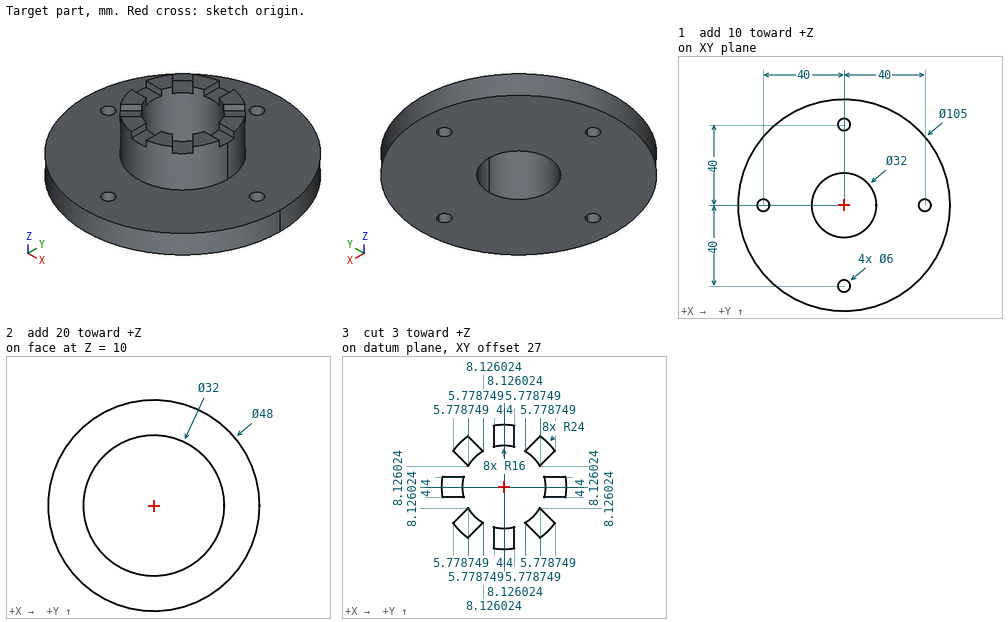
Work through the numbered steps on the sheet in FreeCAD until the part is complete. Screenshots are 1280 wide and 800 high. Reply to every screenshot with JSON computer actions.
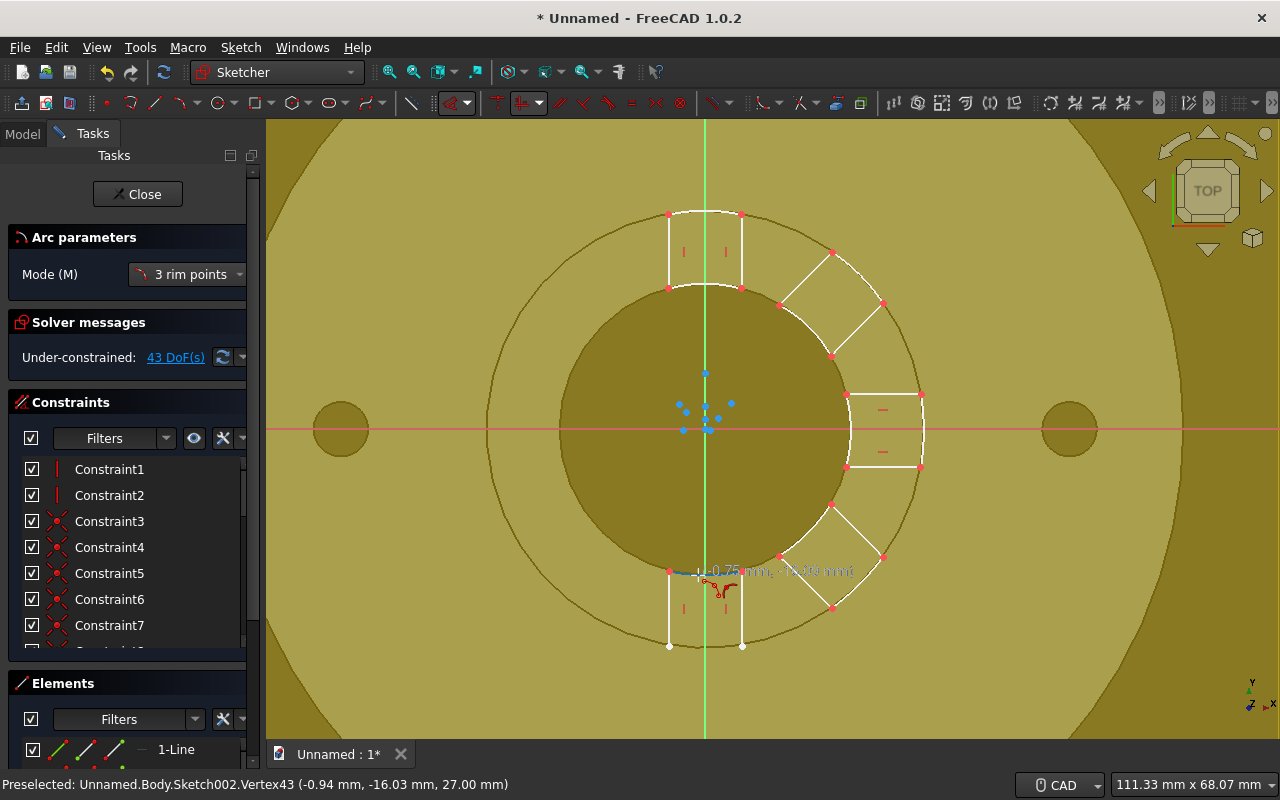
{"action": "left_click", "coordinate": [669, 646]}
{"action": "left_click", "coordinate": [742, 646]}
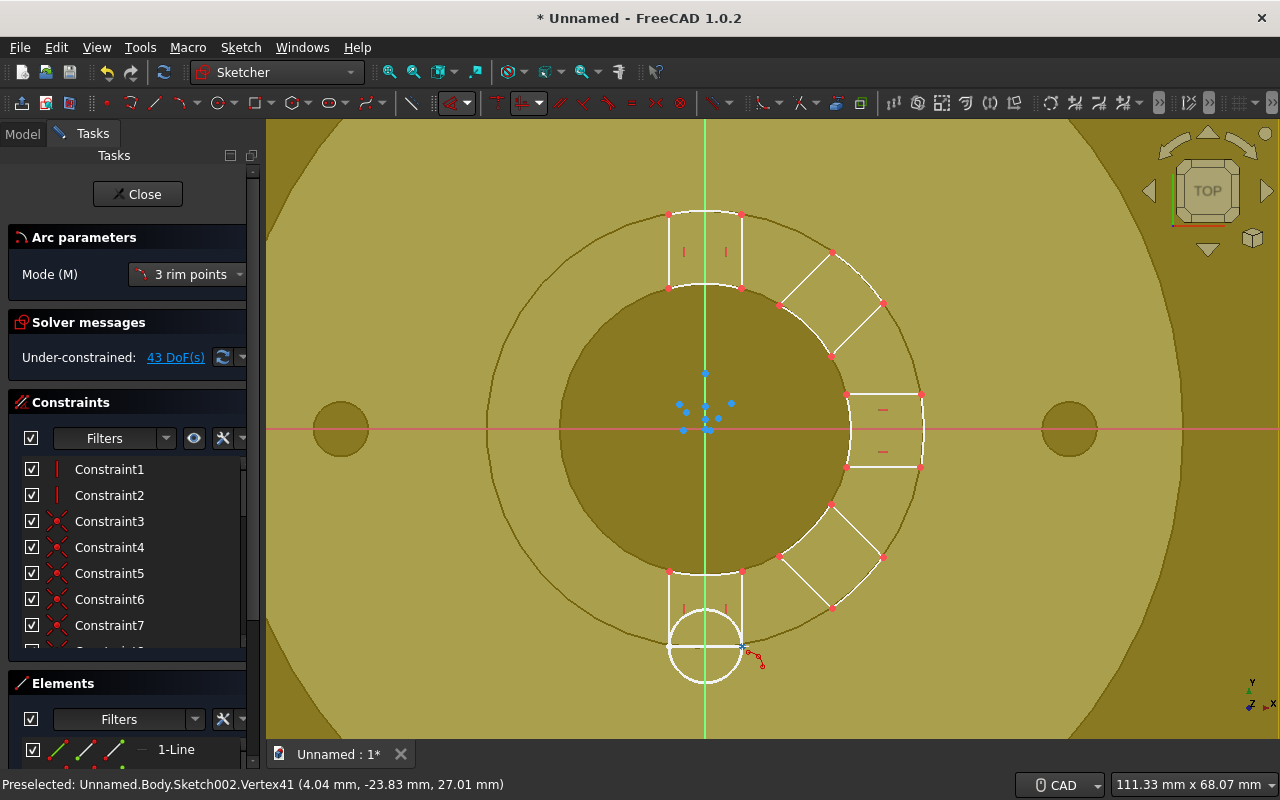
{"action": "scroll", "coordinate": [698, 648], "scroll_direction": "up", "scroll_amount": 9}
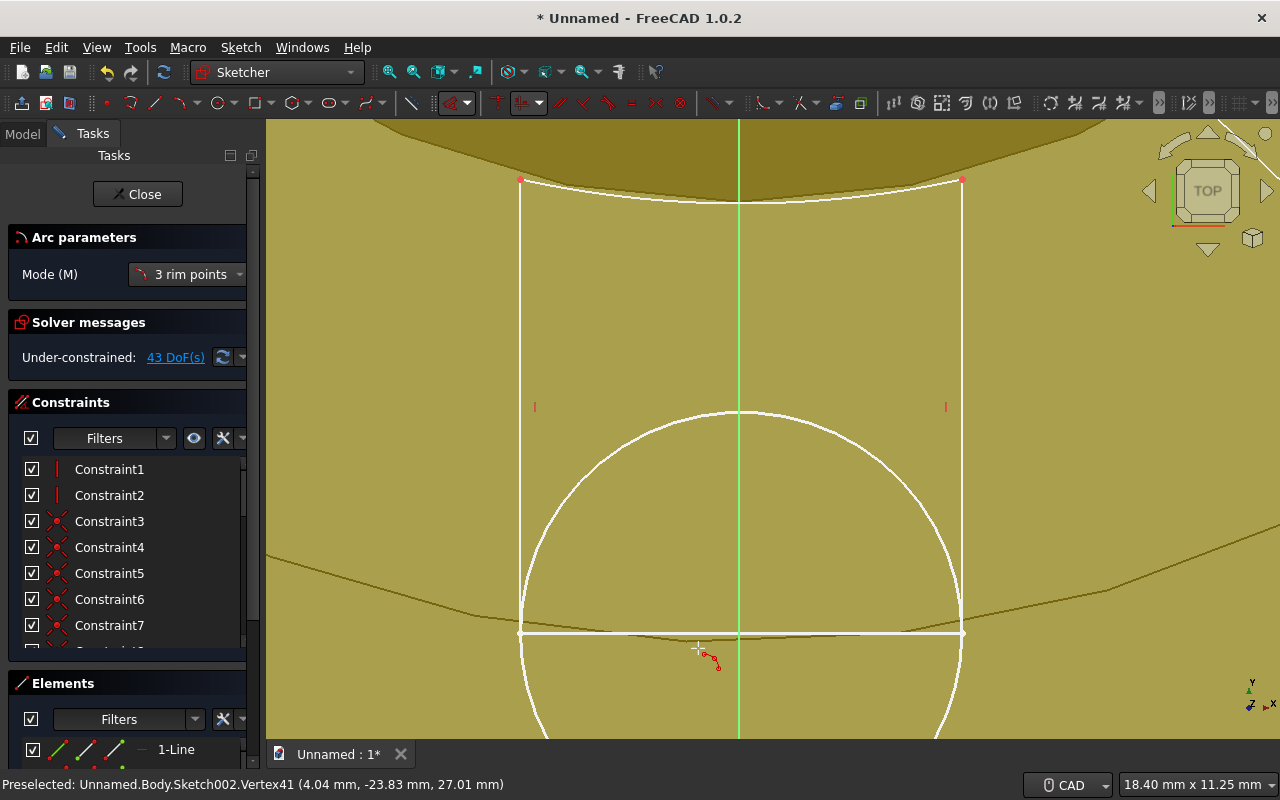
{"action": "left_click", "coordinate": [695, 642]}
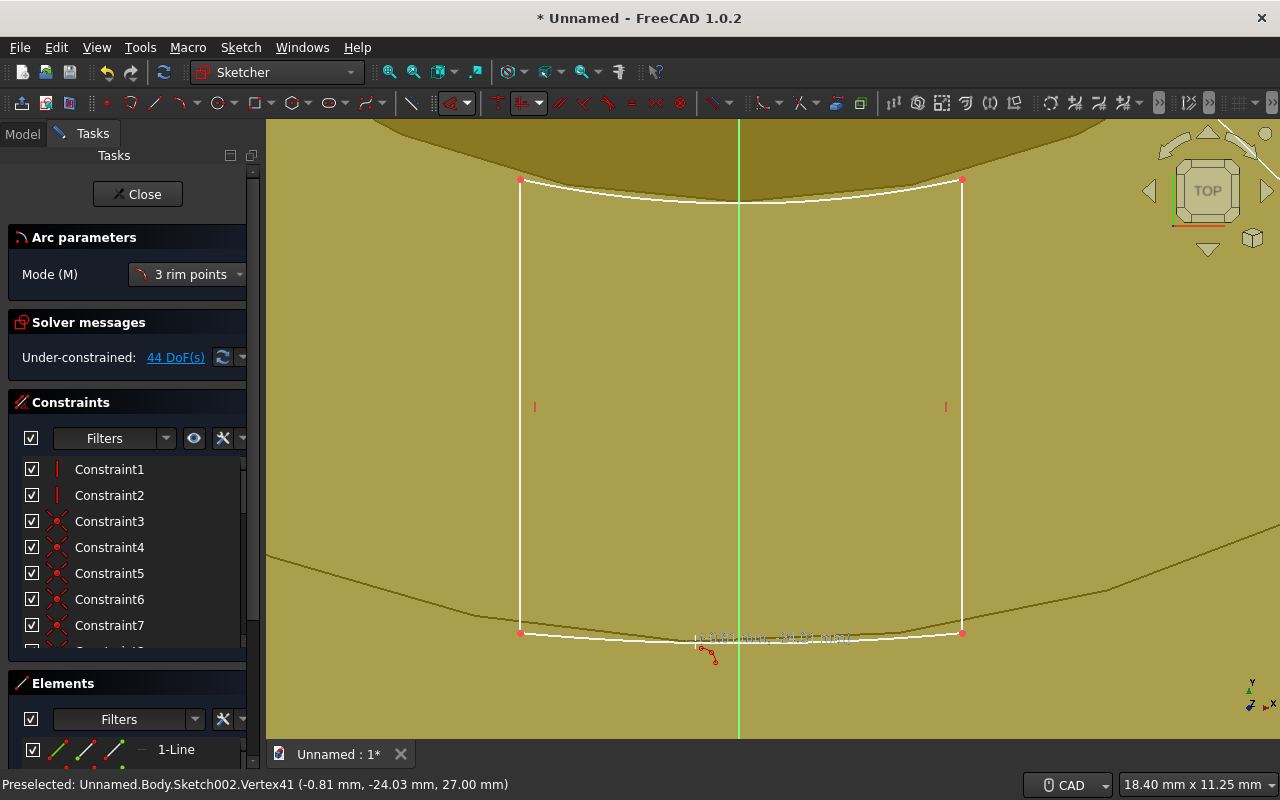
{"action": "left_click", "coordinate": [156, 104]}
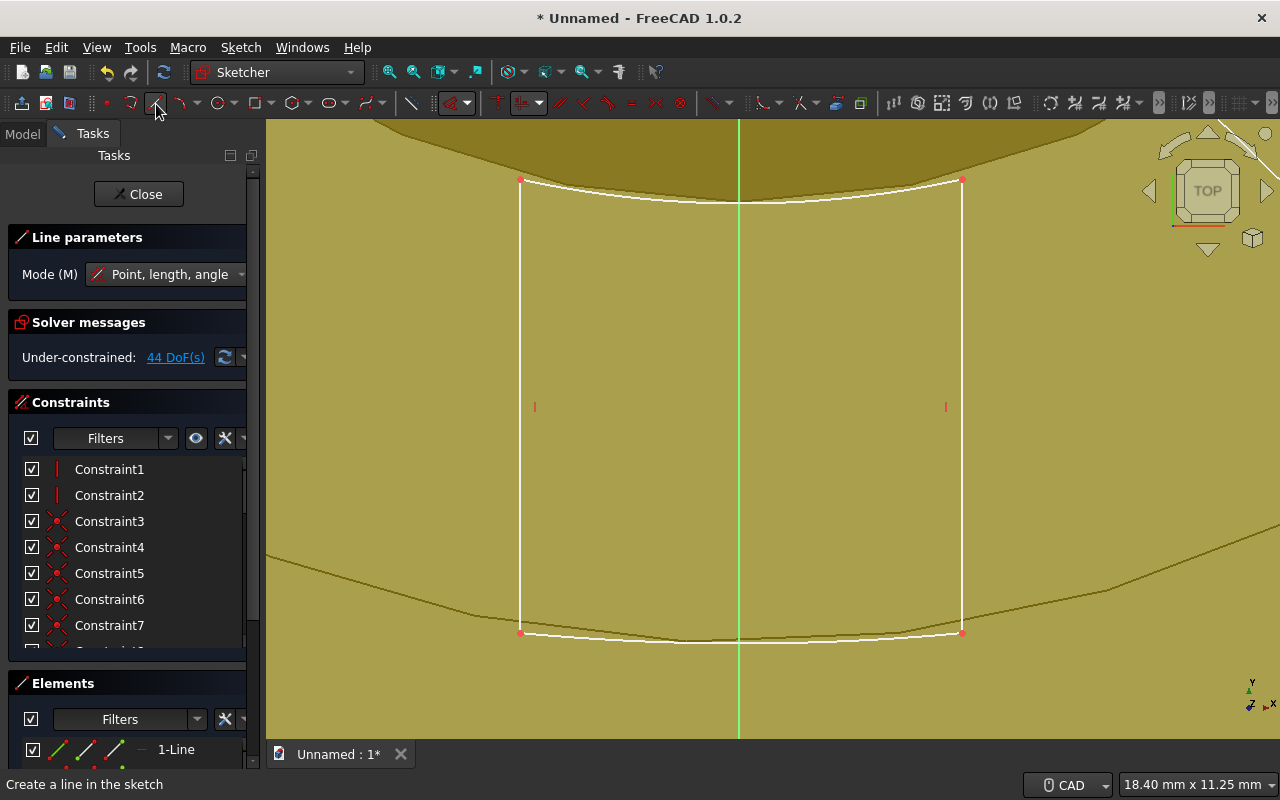
{"action": "scroll", "coordinate": [698, 649], "scroll_direction": "down", "scroll_amount": 9}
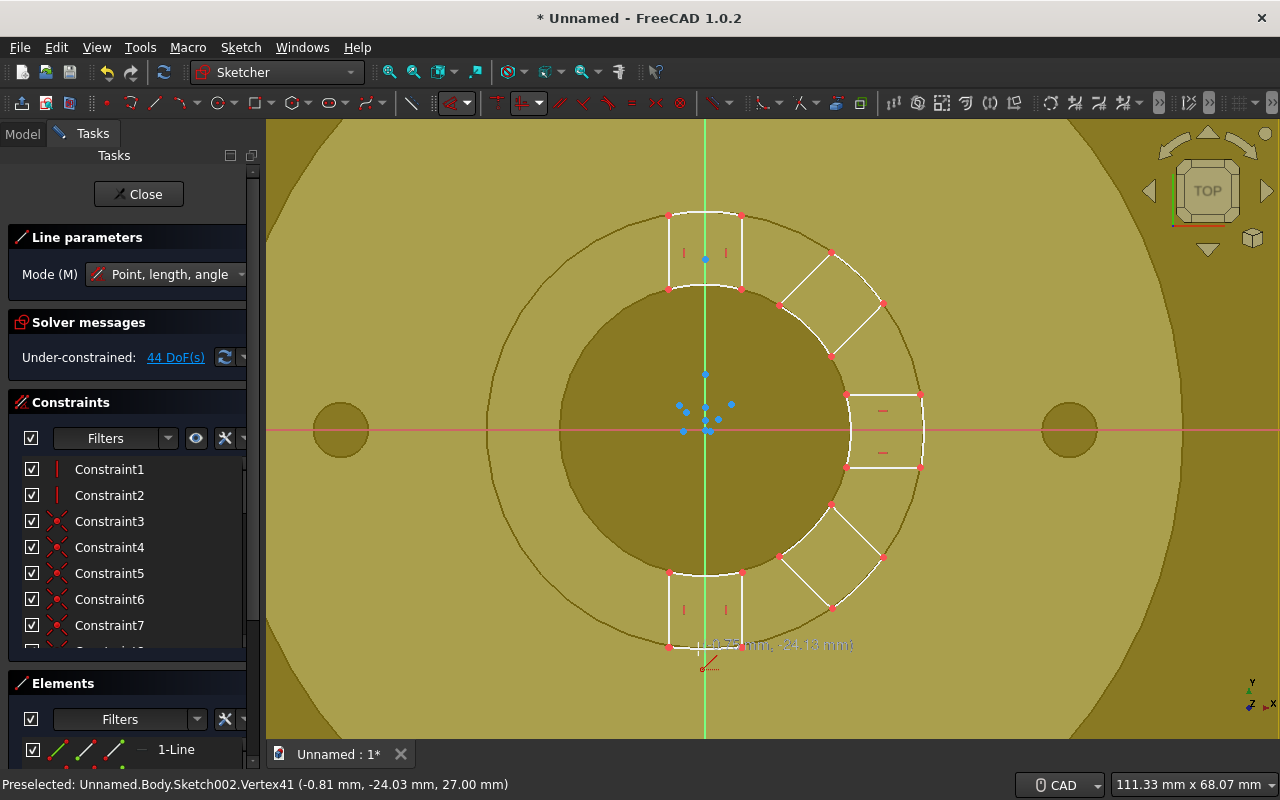
{"action": "left_click", "coordinate": [579, 608]}
{"action": "left_click", "coordinate": [631, 556]}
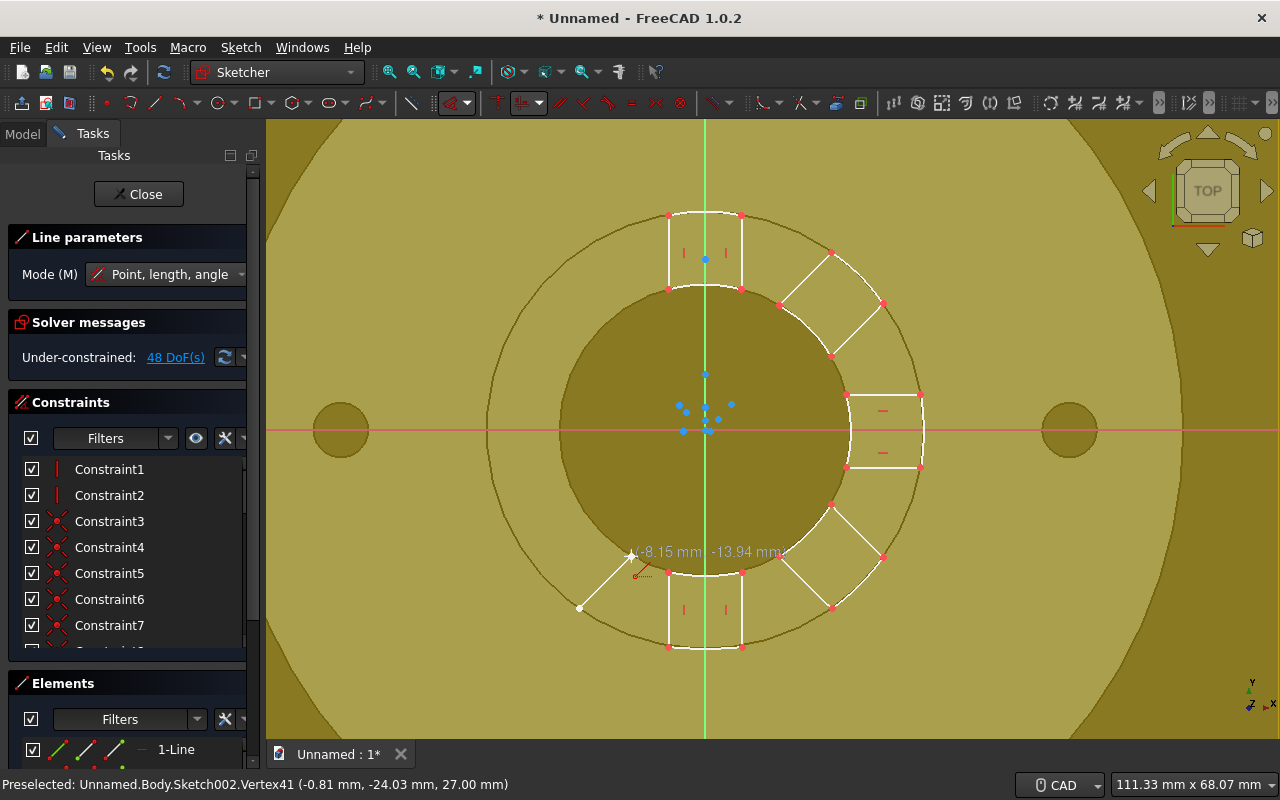
{"action": "left_click", "coordinate": [580, 504]}
{"action": "left_click", "coordinate": [527, 557]}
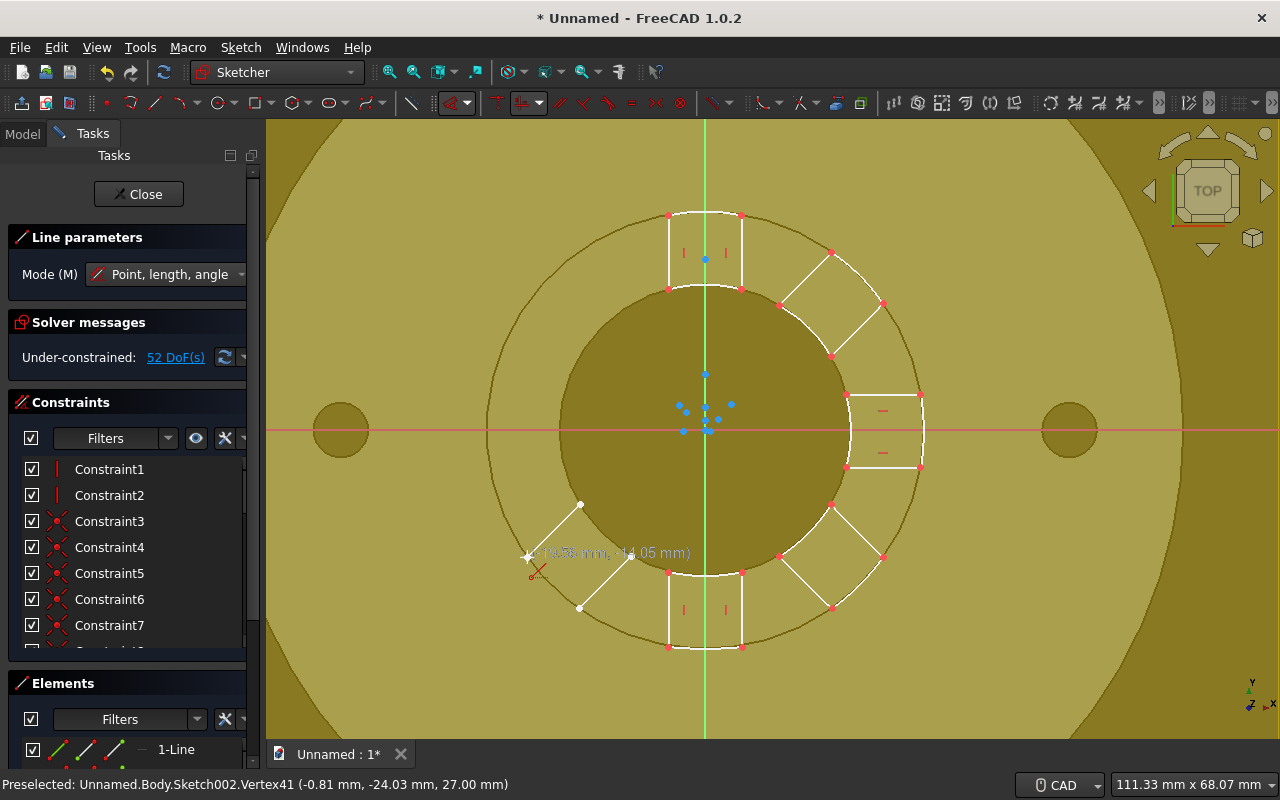
{"action": "left_click", "coordinate": [180, 104]}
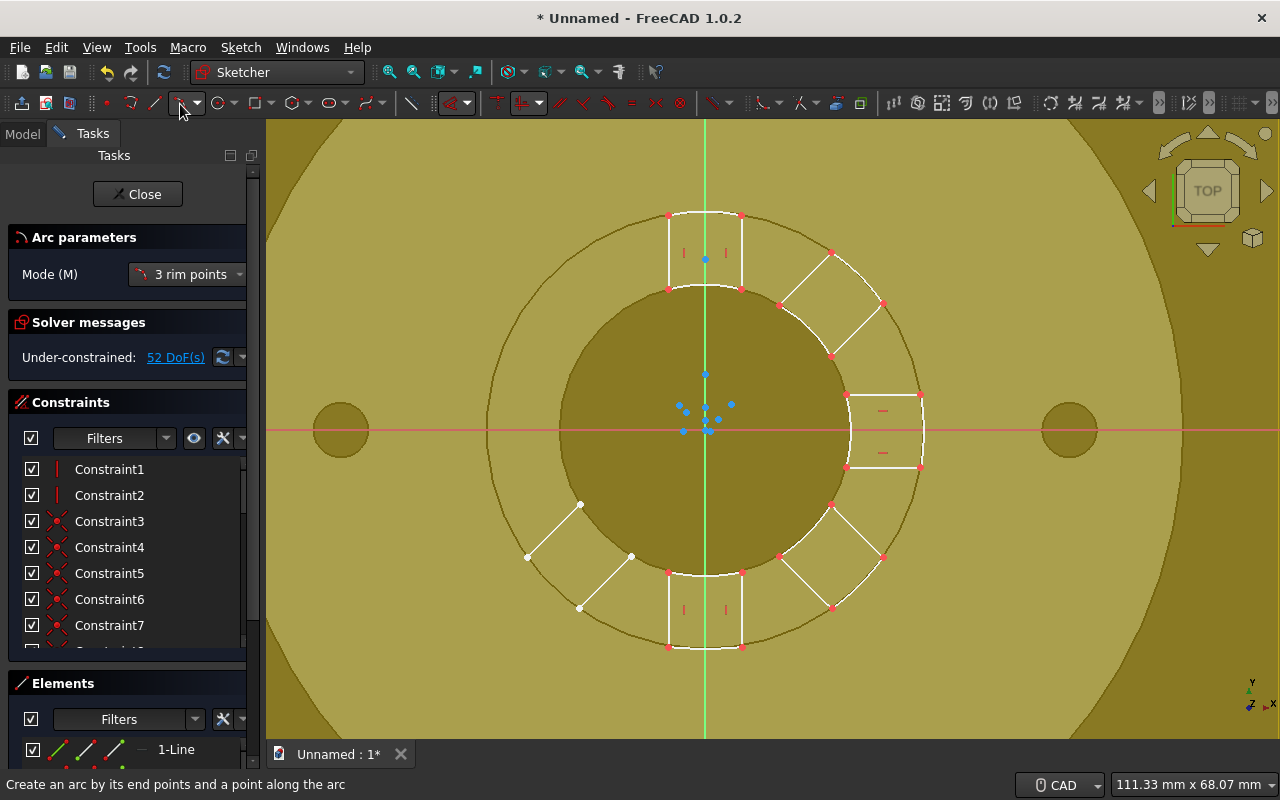
{"action": "left_click", "coordinate": [631, 557]}
{"action": "left_click", "coordinate": [580, 505]}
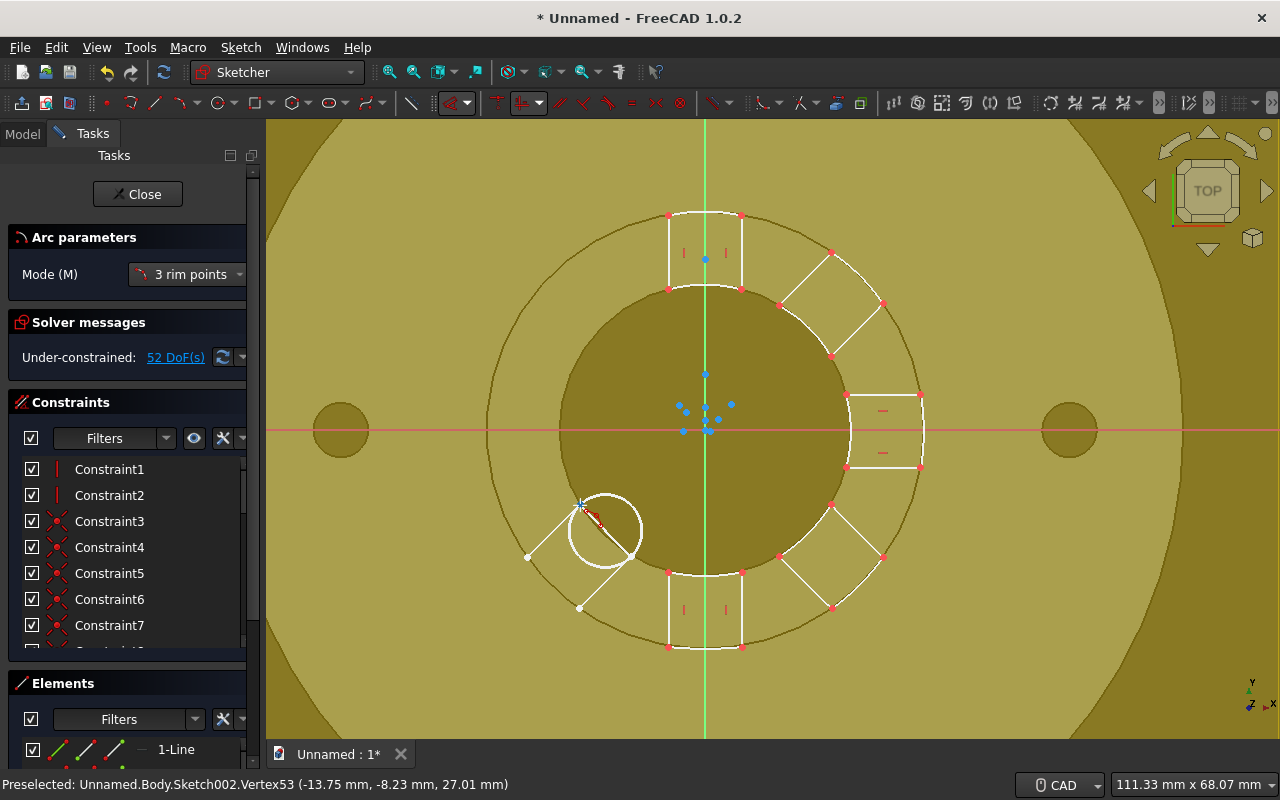
{"action": "scroll", "coordinate": [602, 533], "scroll_direction": "up", "scroll_amount": 7}